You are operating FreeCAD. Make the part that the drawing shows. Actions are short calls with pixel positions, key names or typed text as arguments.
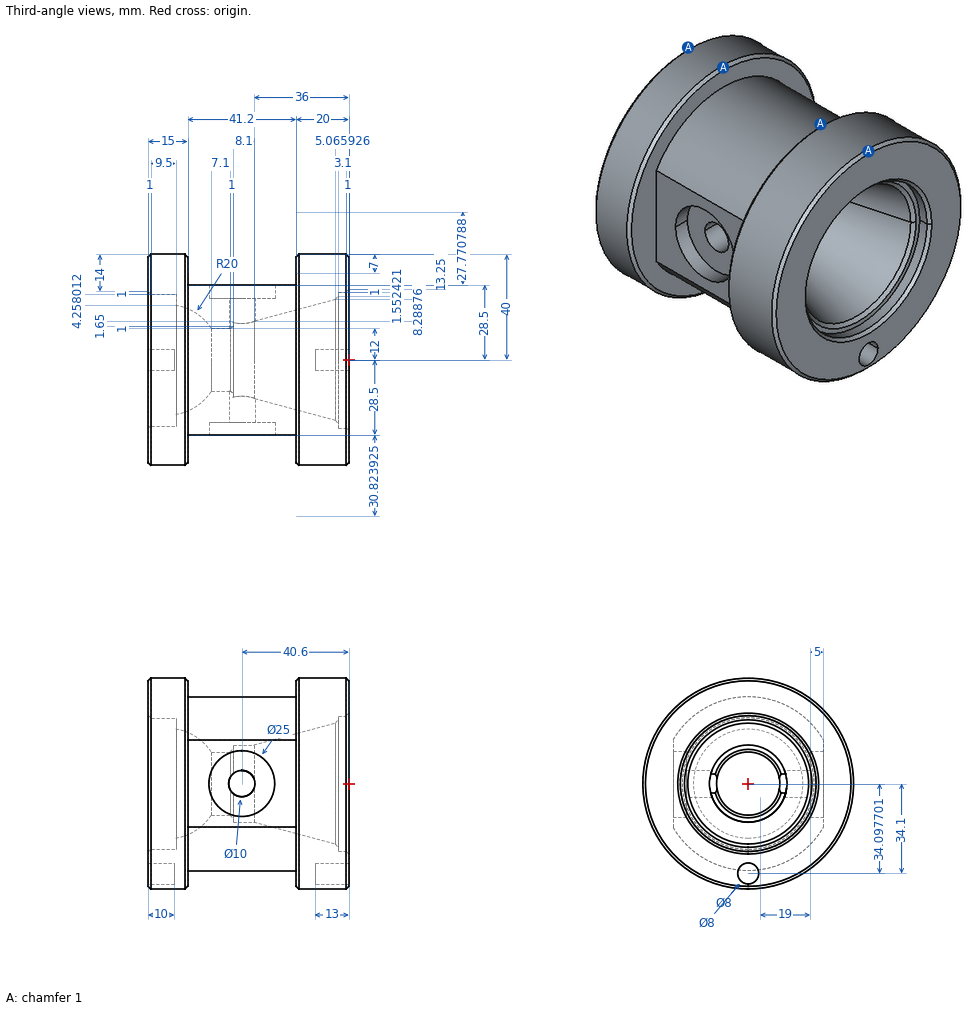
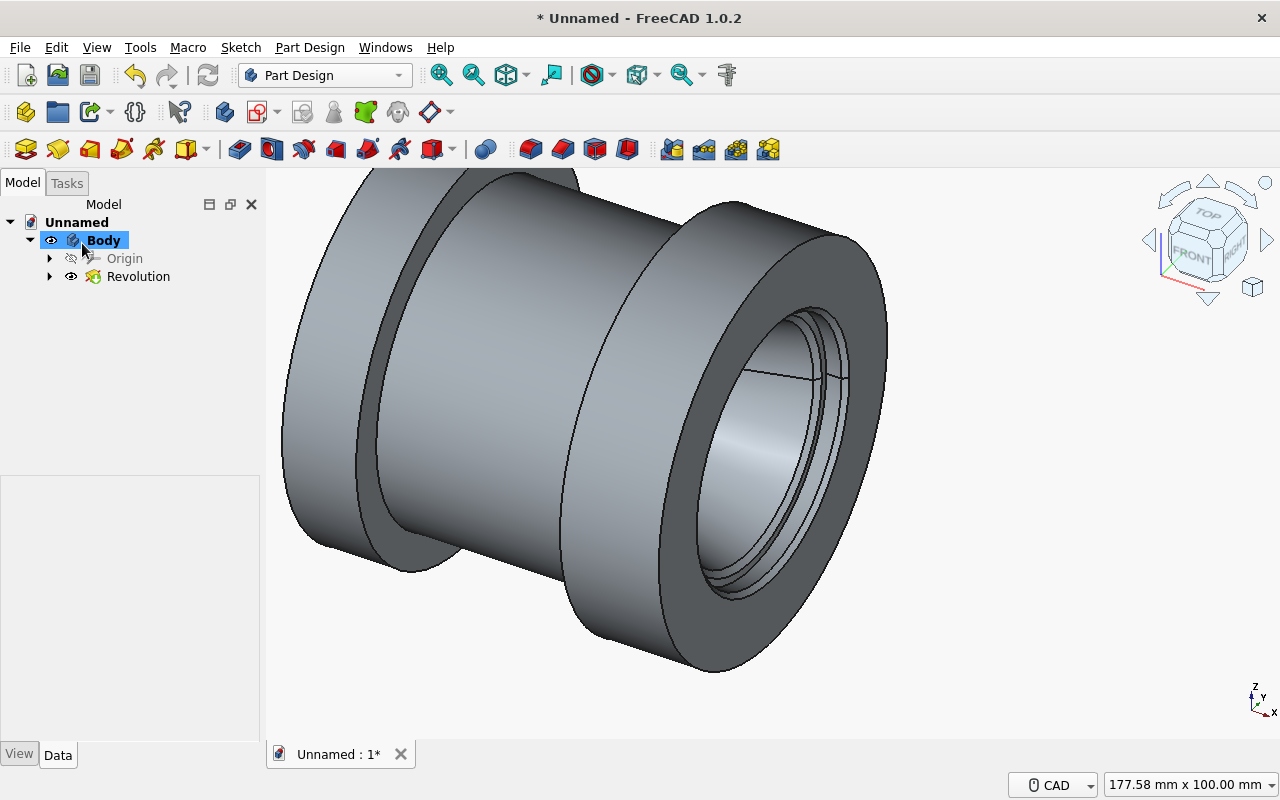
click(442, 76)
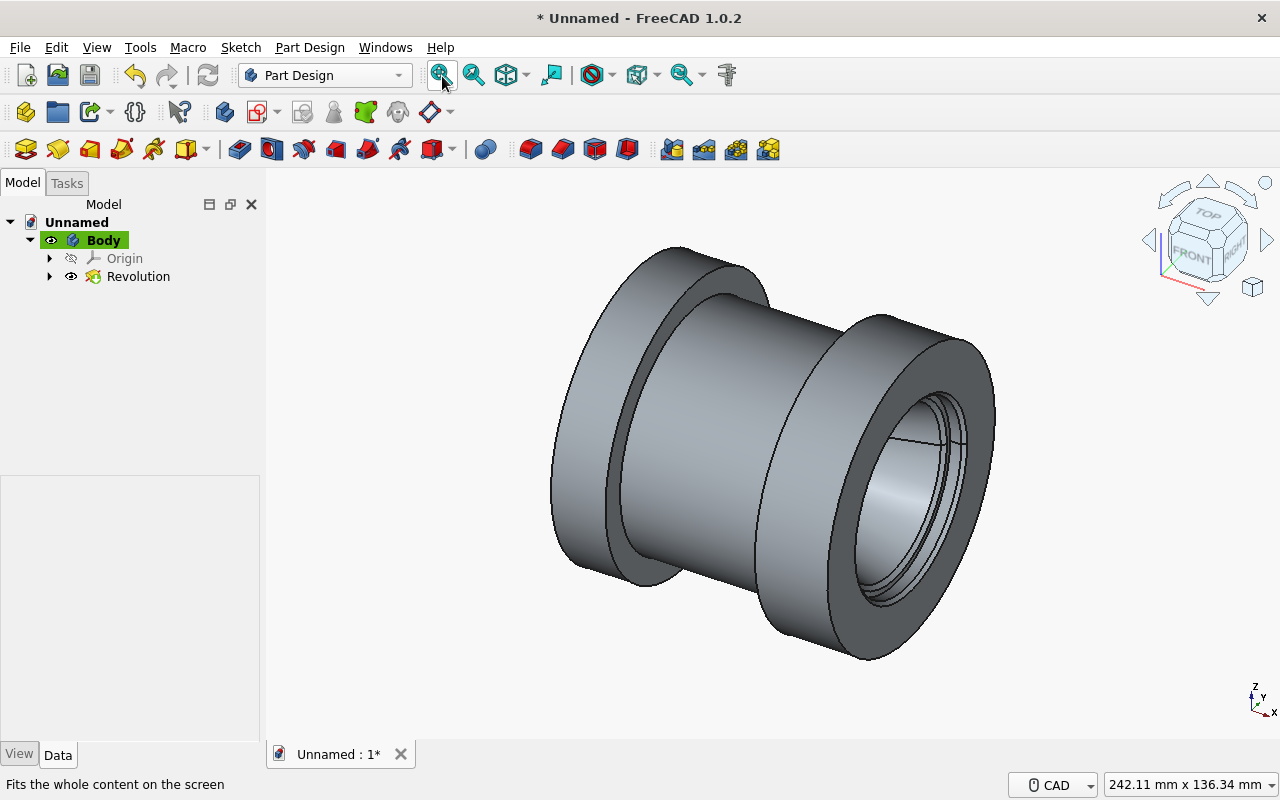
click(827, 582)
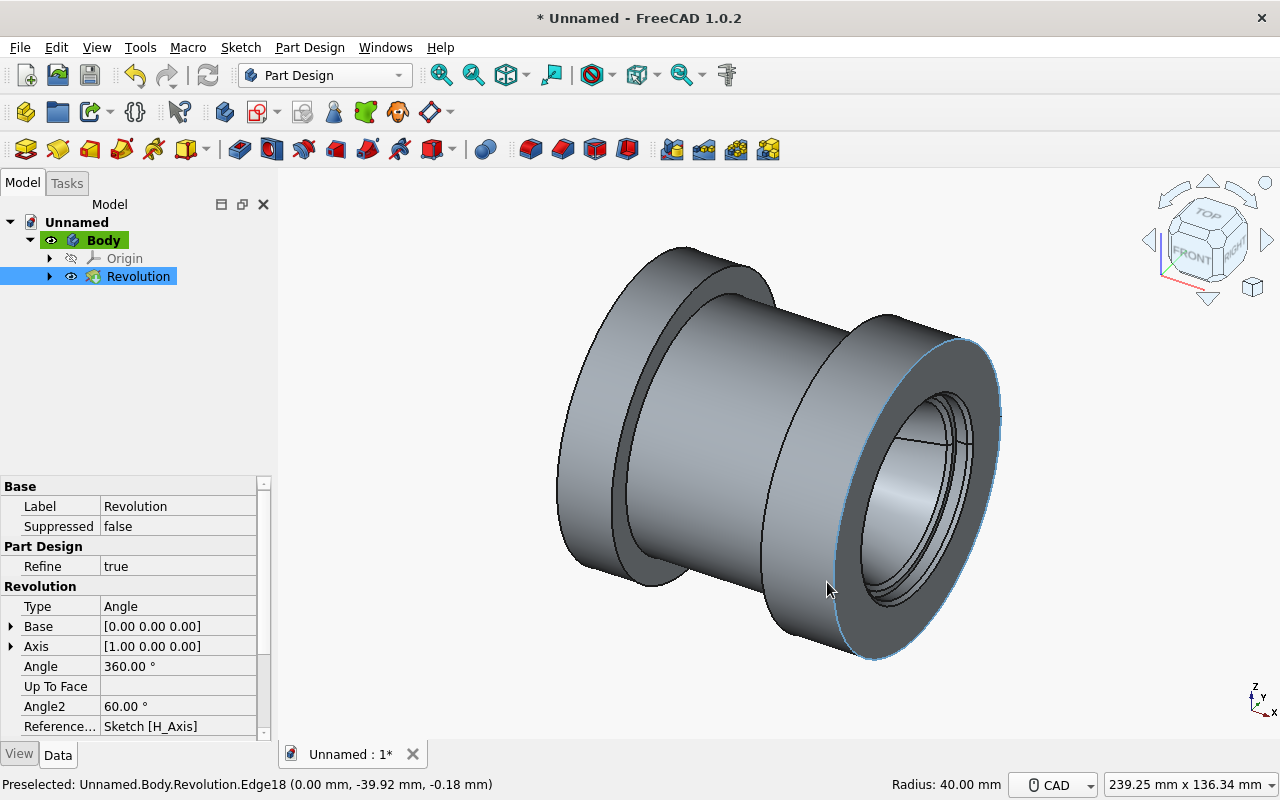
click(611, 508, ctrl)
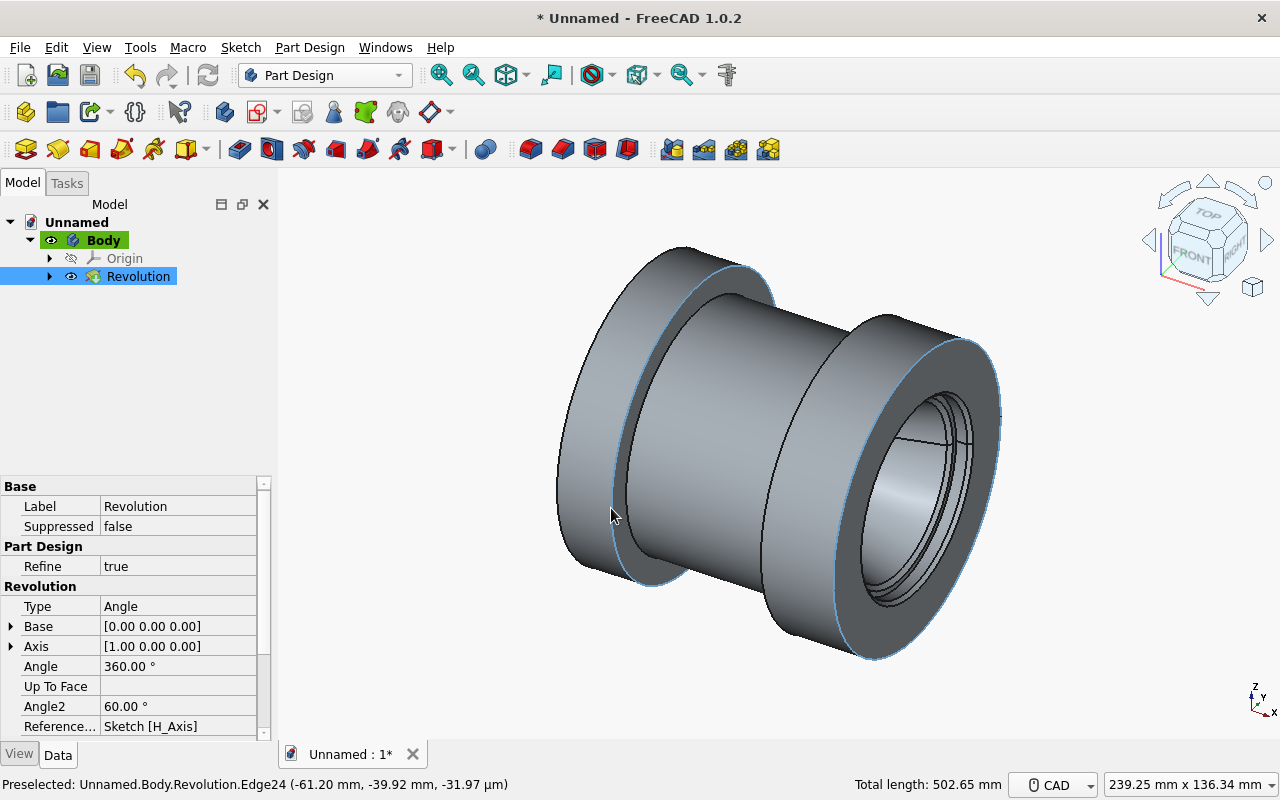
key(0)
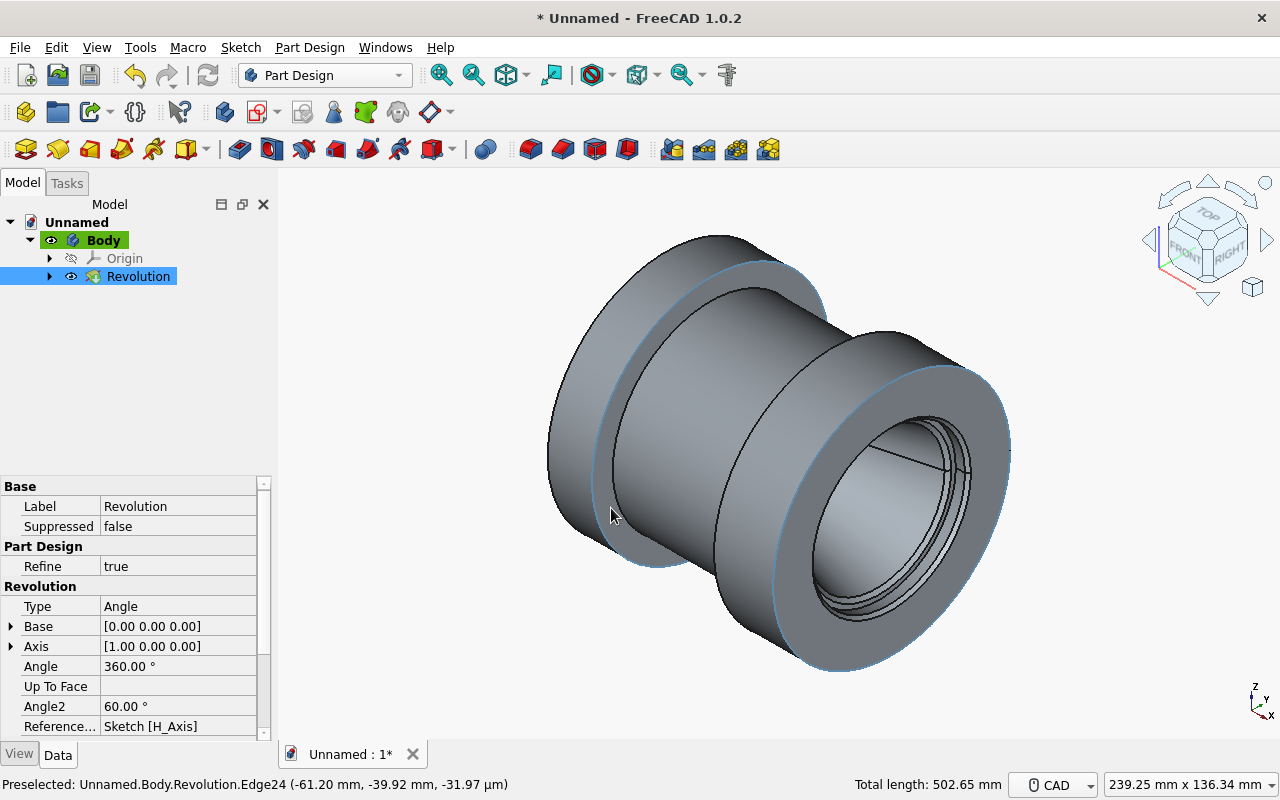
key(2)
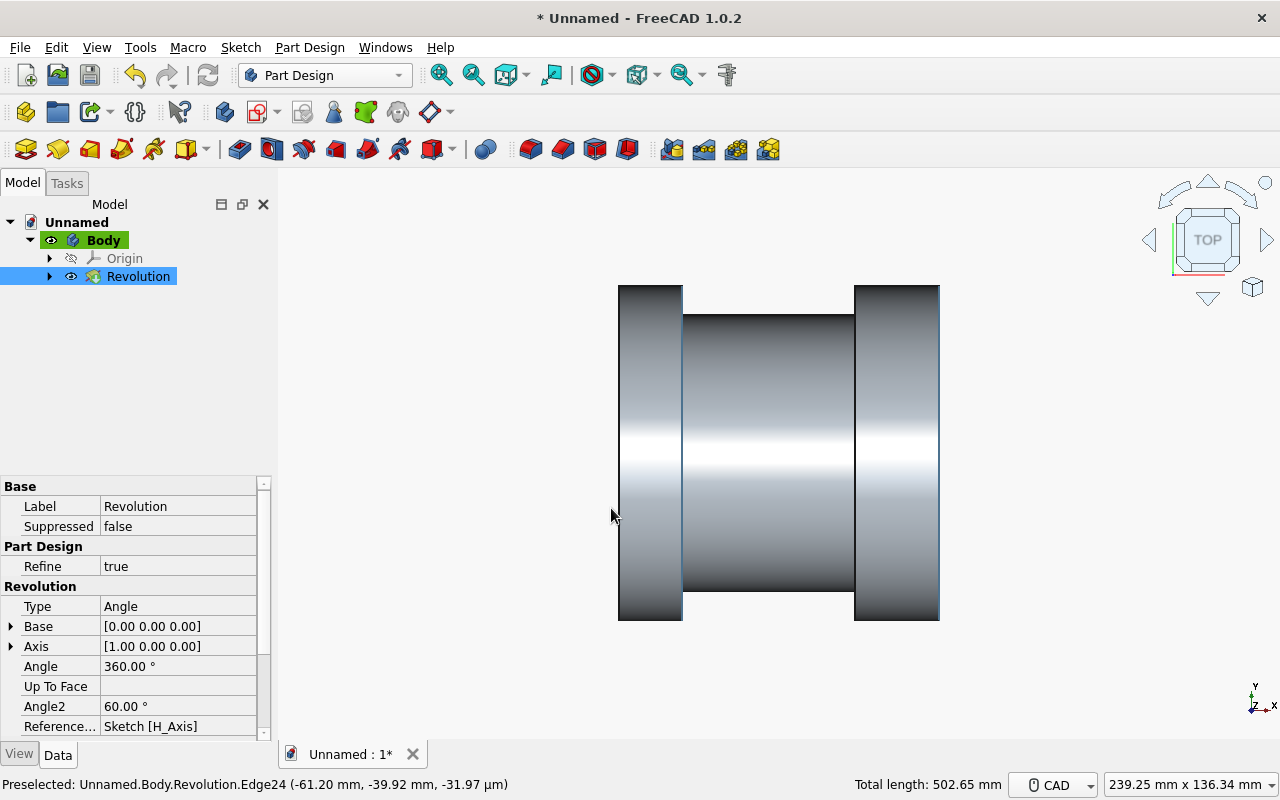
click(855, 588, ctrl)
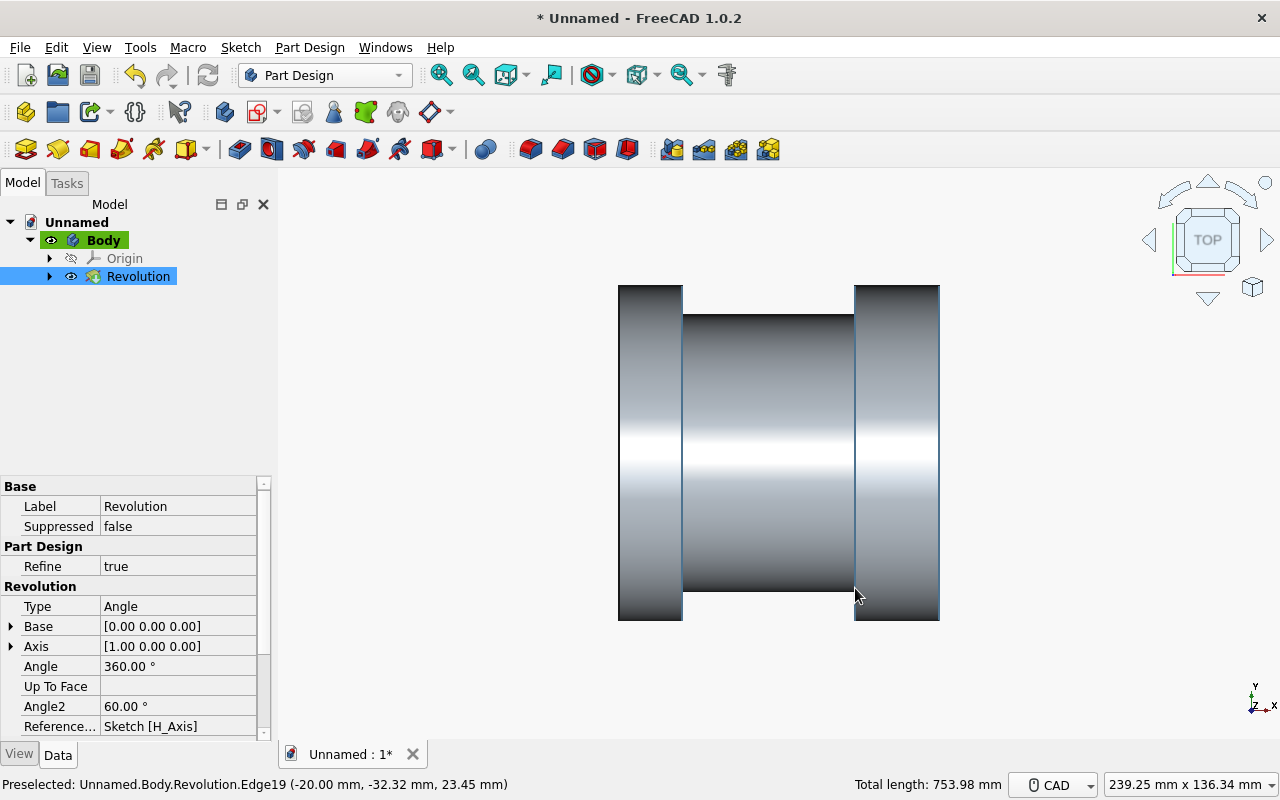
click(619, 588, ctrl)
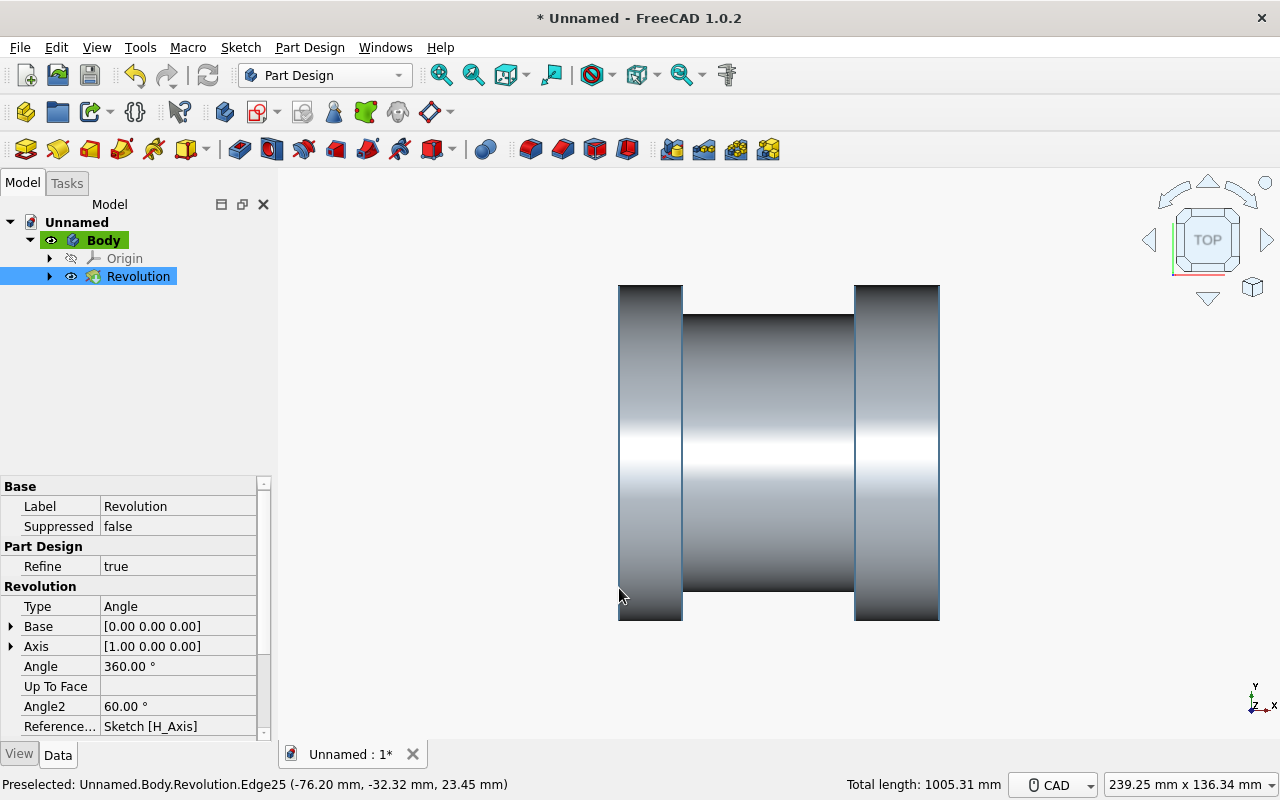
click(564, 150)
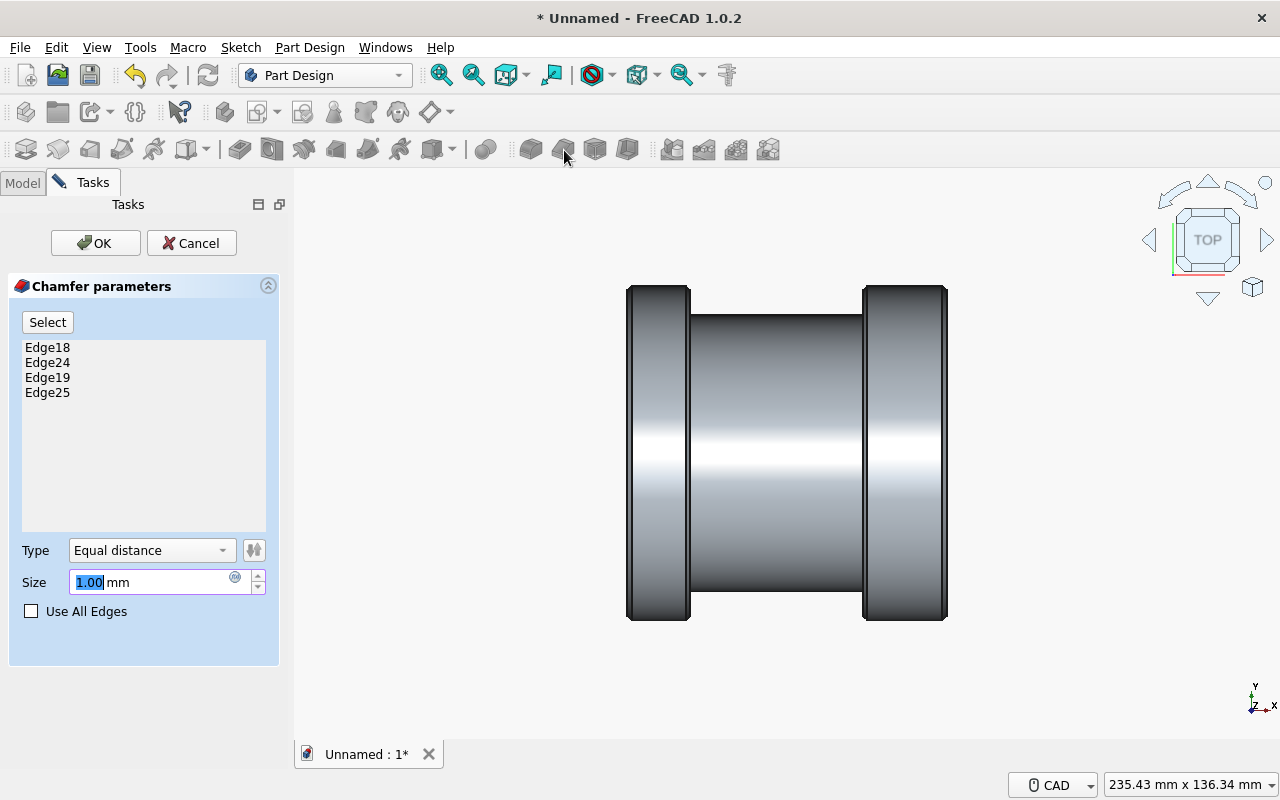
text(1)
key(Tab)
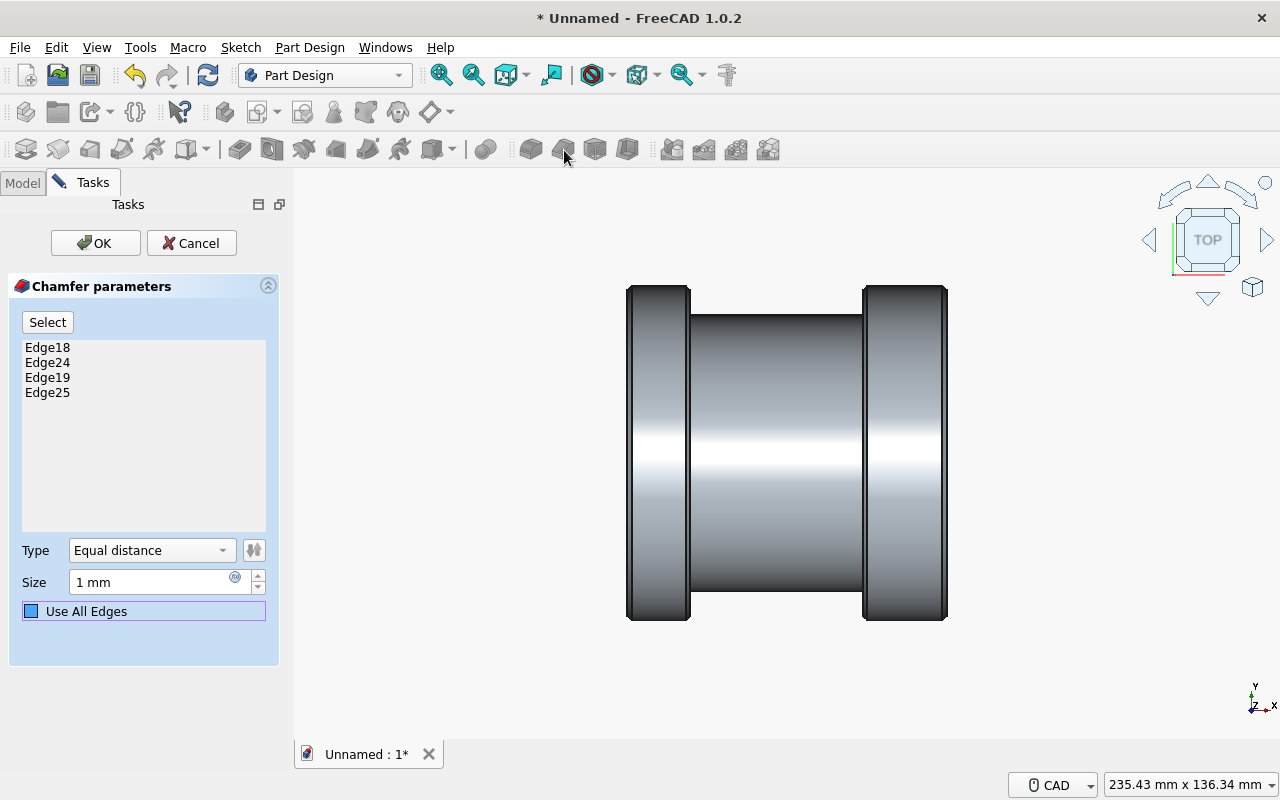
click(96, 243)